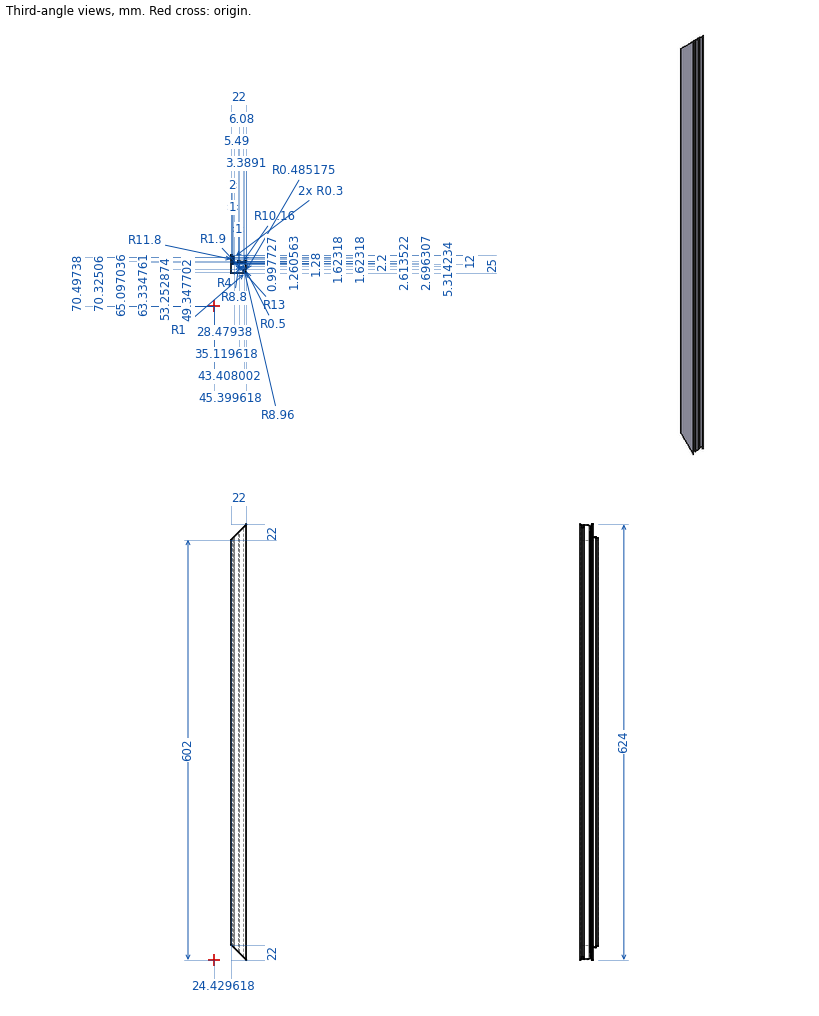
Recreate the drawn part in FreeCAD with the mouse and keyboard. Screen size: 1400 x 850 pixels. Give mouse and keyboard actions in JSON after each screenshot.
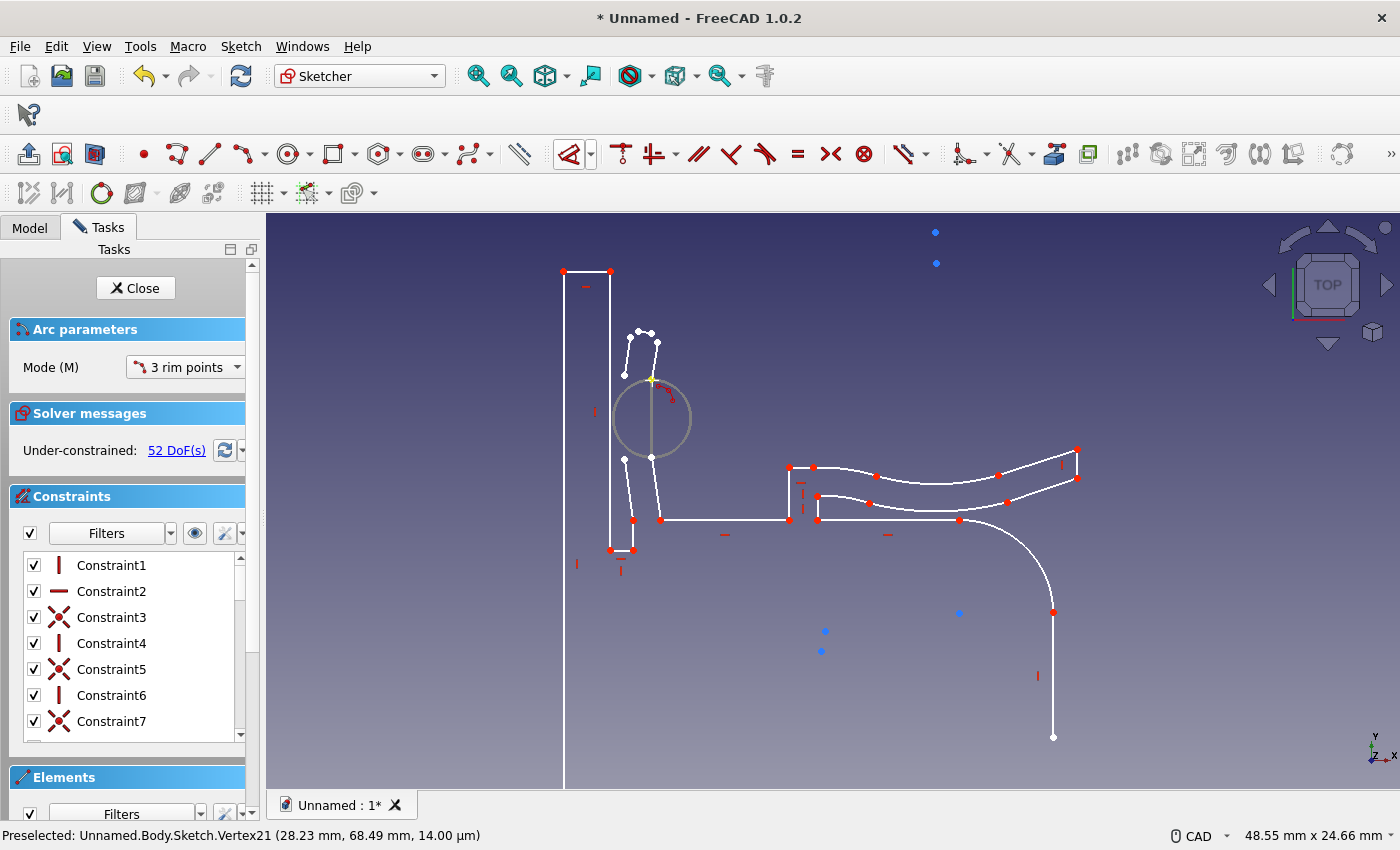
{"action": "scroll", "coordinate": [650, 417], "scroll_direction": "up", "scroll_amount": 9}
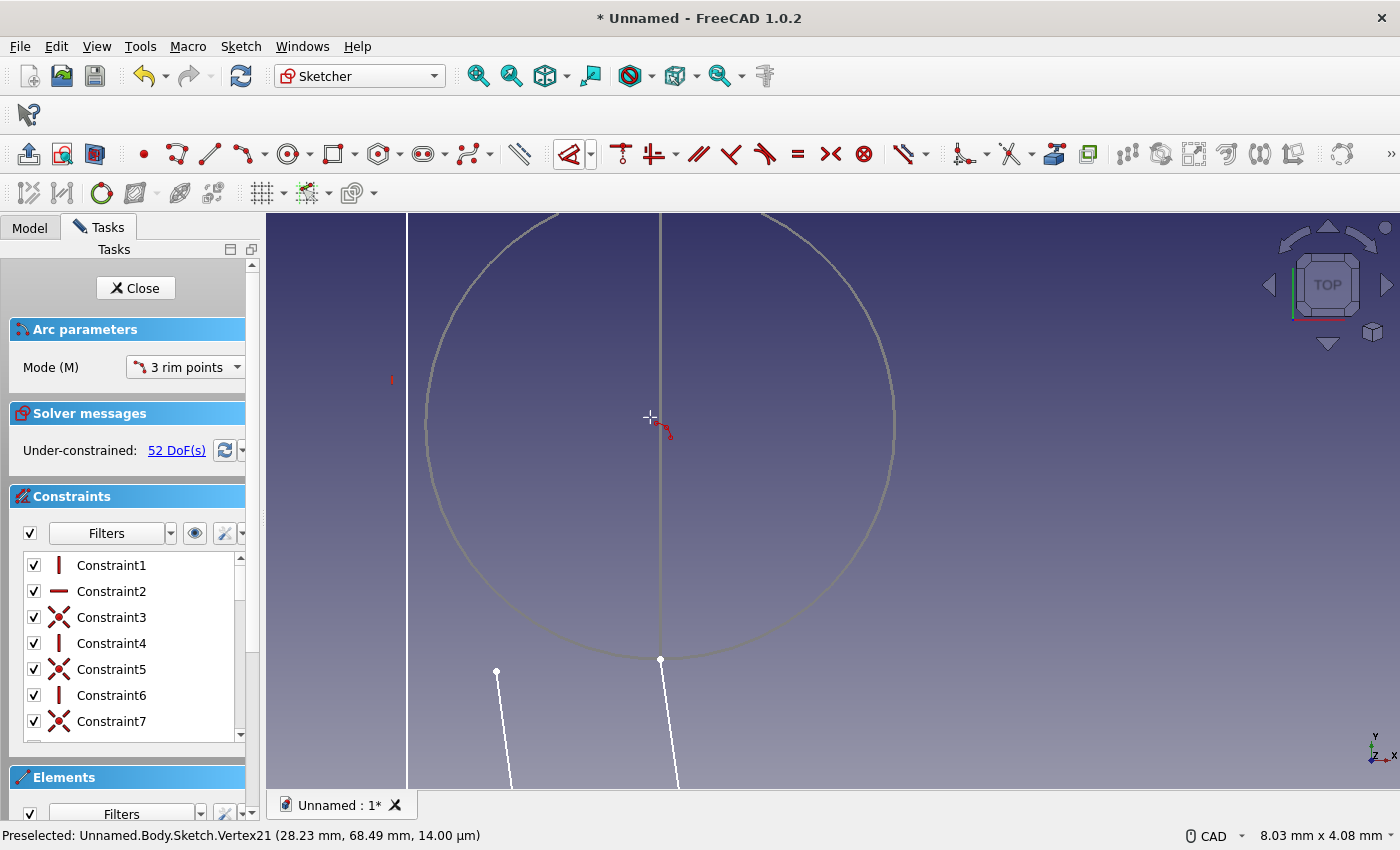
{"action": "left_click", "coordinate": [648, 415]}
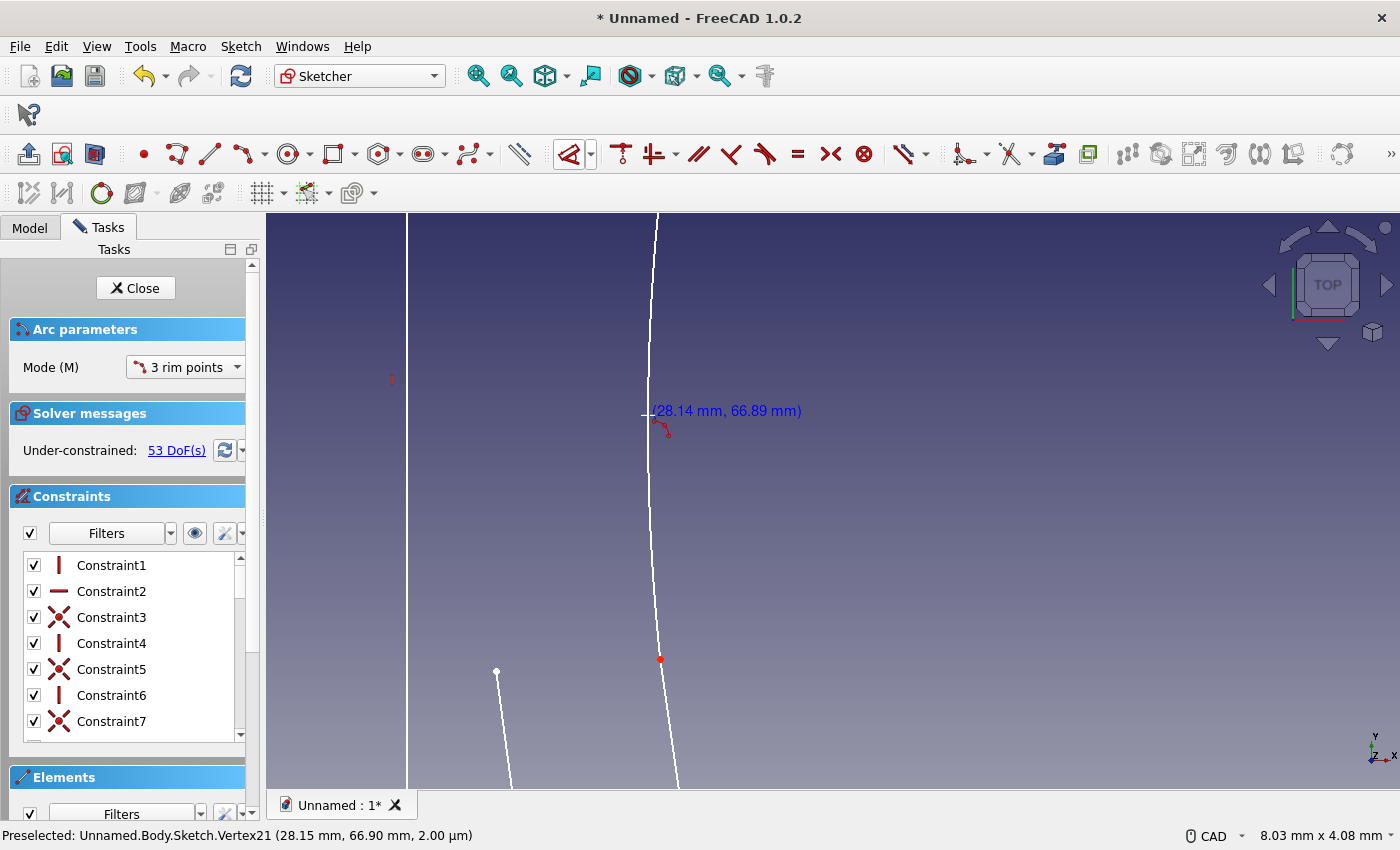
{"action": "scroll", "coordinate": [651, 403], "scroll_direction": "down", "scroll_amount": 11}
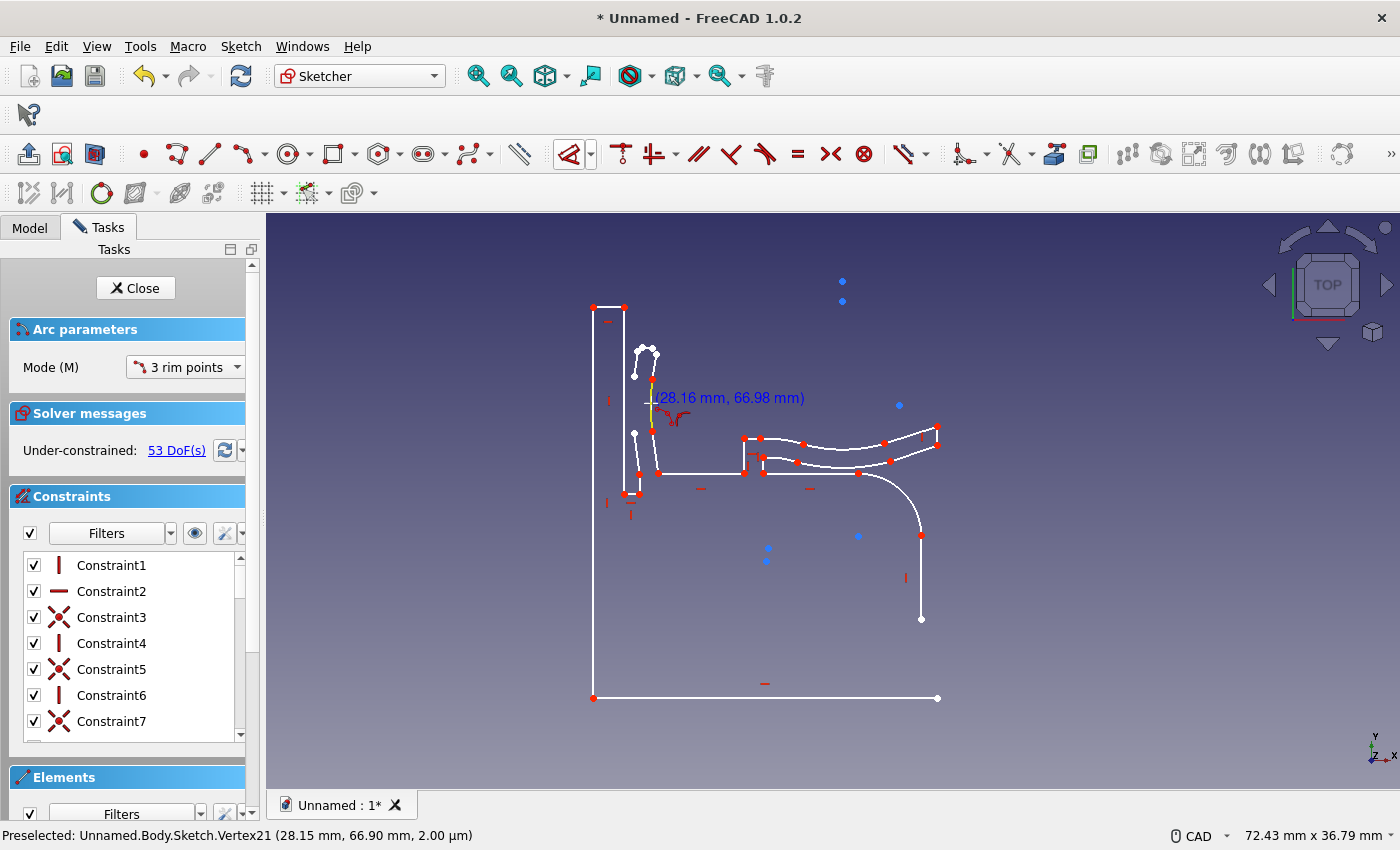
{"action": "scroll", "coordinate": [656, 354], "scroll_direction": "up", "scroll_amount": 5}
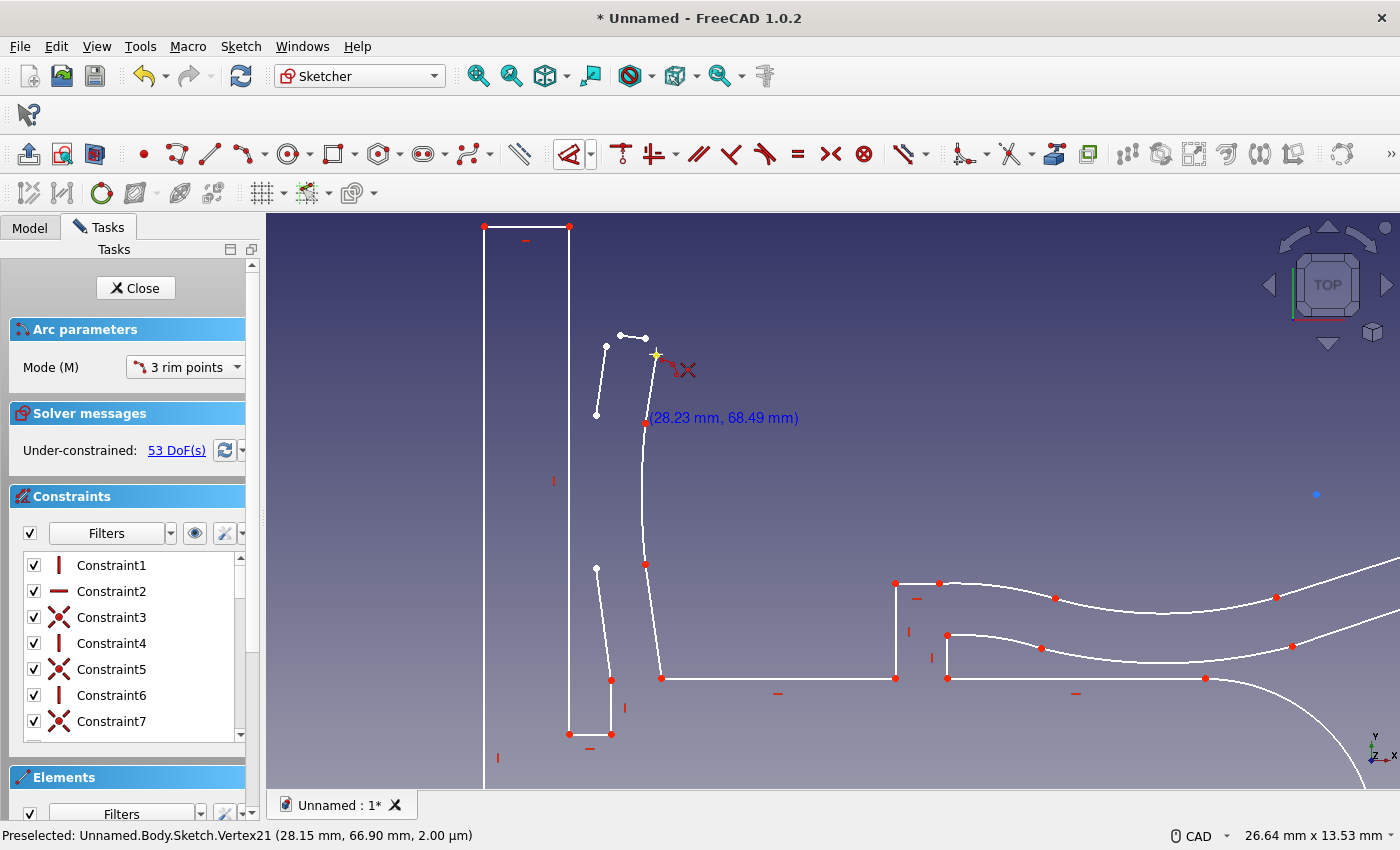
{"action": "left_click", "coordinate": [656, 355]}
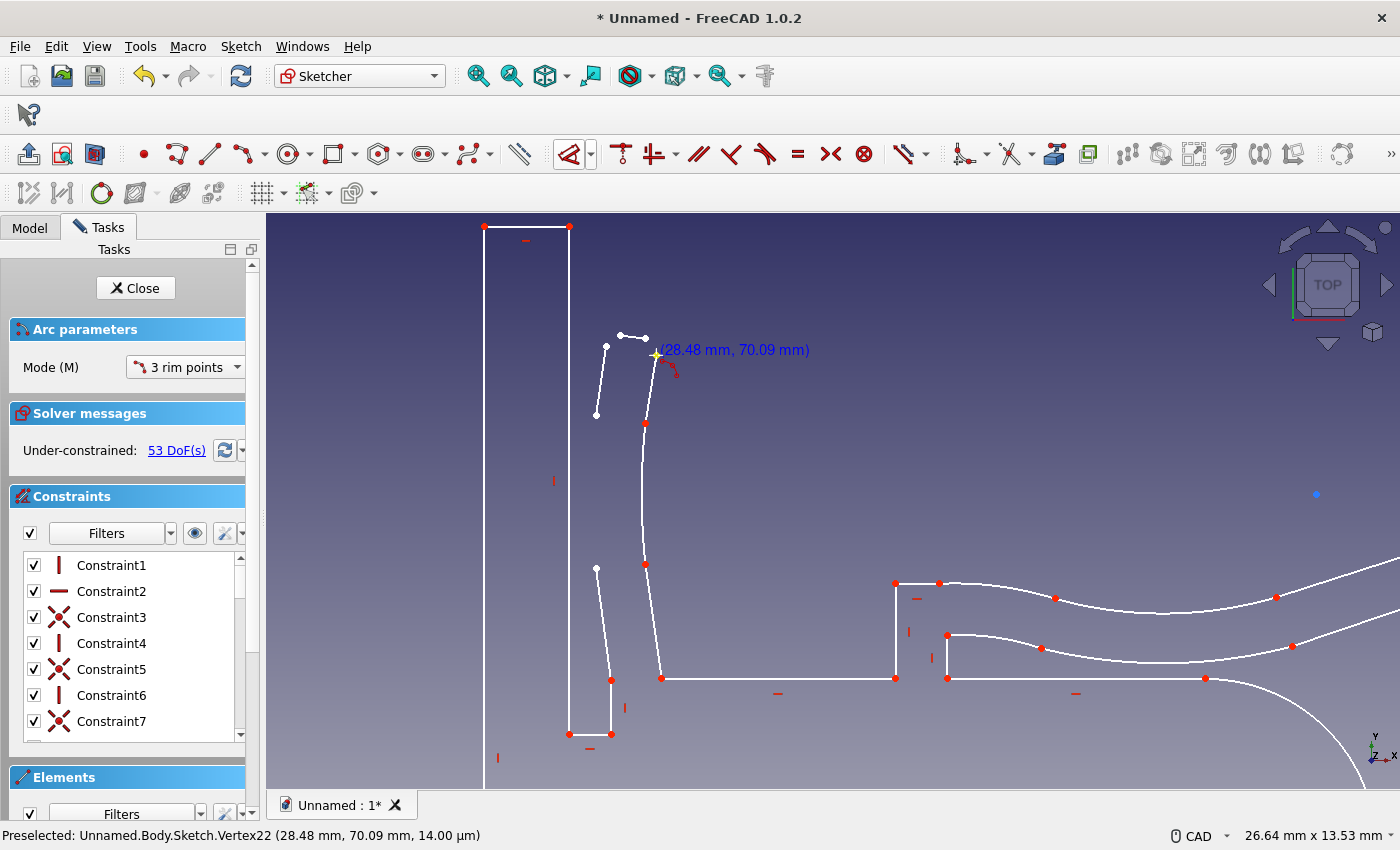
{"action": "scroll", "coordinate": [645, 338], "scroll_direction": "up", "scroll_amount": 2}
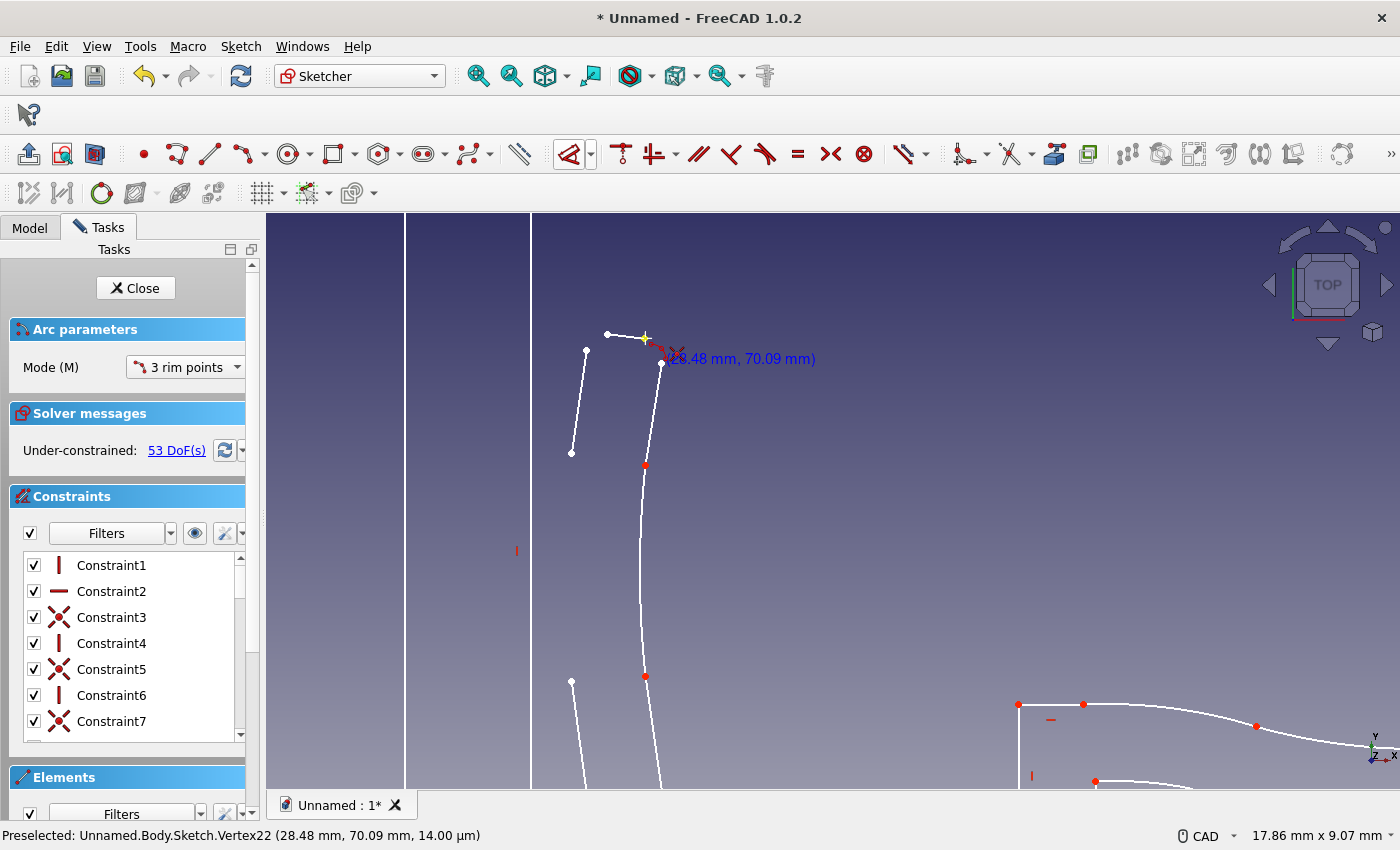
{"action": "left_click", "coordinate": [645, 339]}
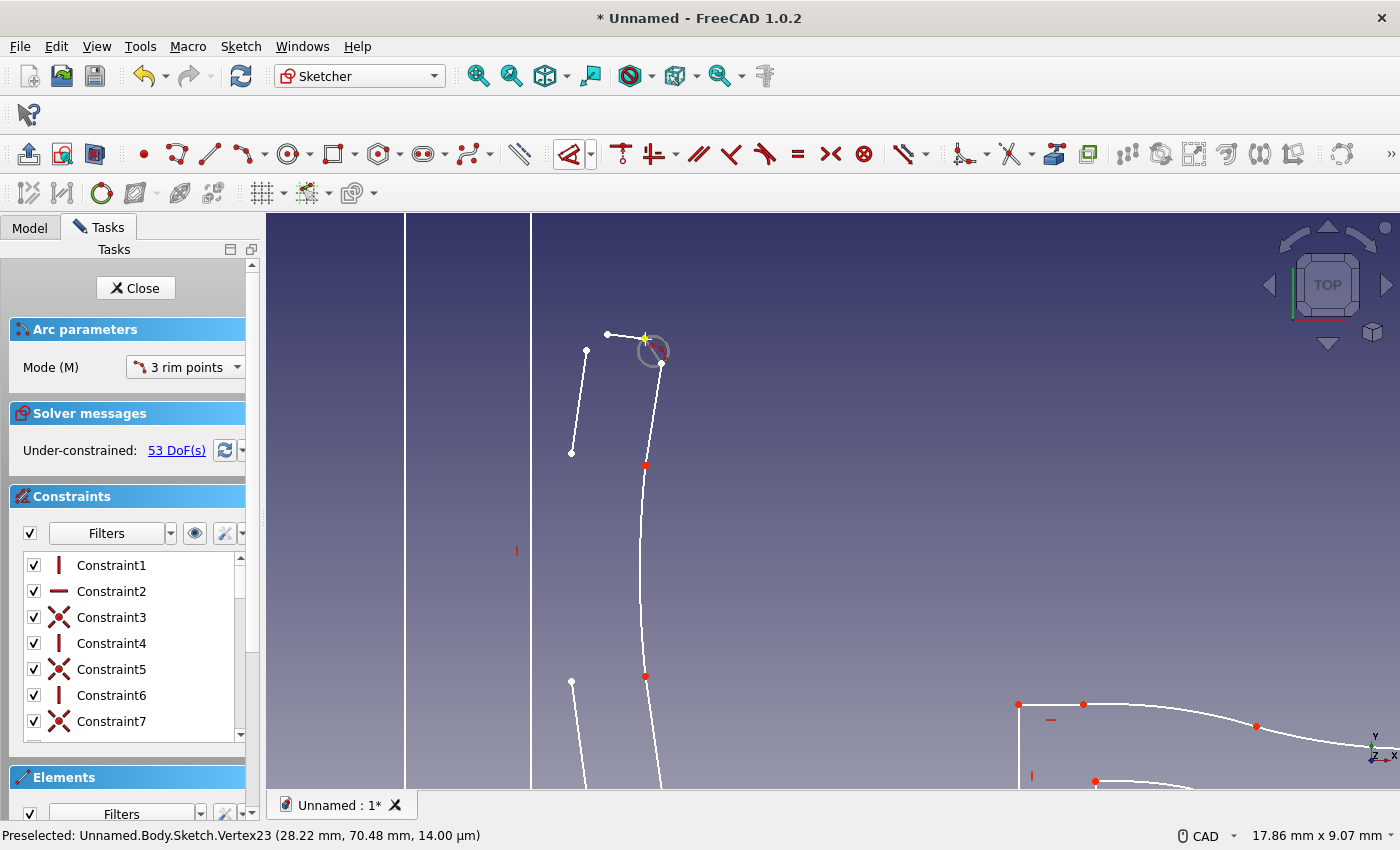
{"action": "scroll", "coordinate": [658, 345], "scroll_direction": "up", "scroll_amount": 6}